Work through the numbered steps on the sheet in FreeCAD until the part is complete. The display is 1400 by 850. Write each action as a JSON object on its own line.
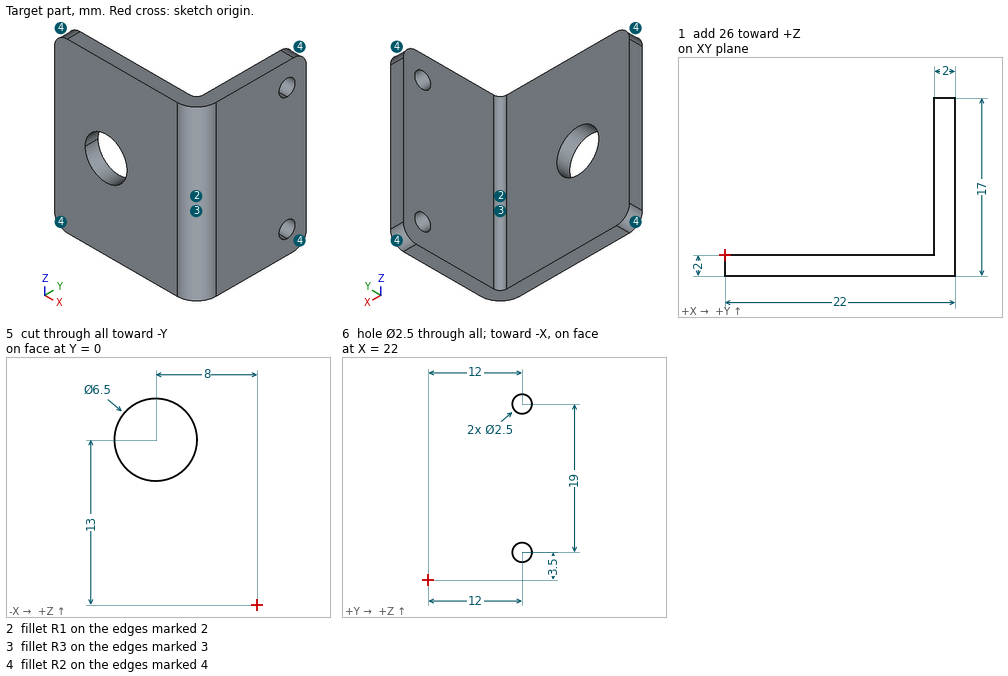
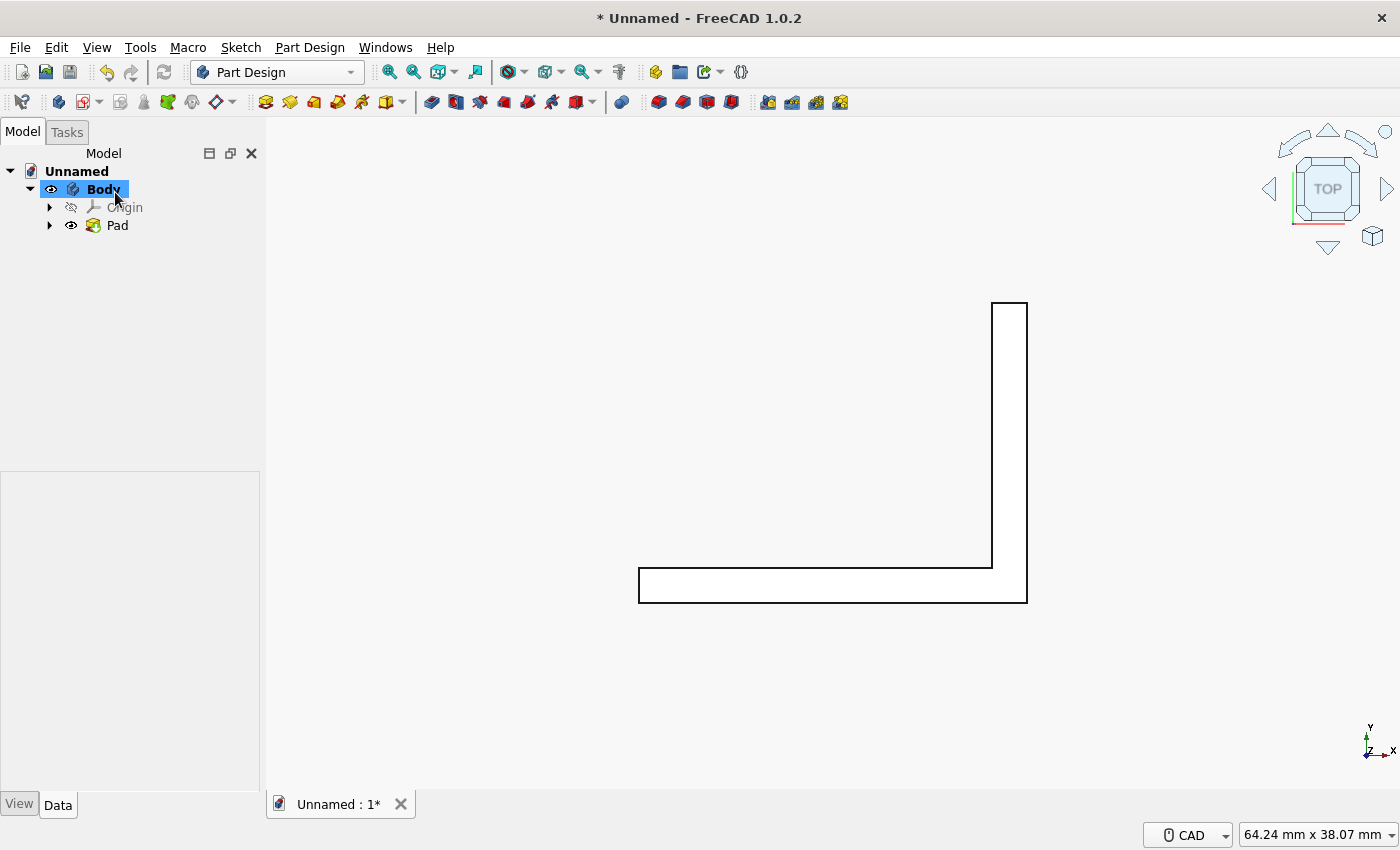
{"action": "key", "text": "v f"}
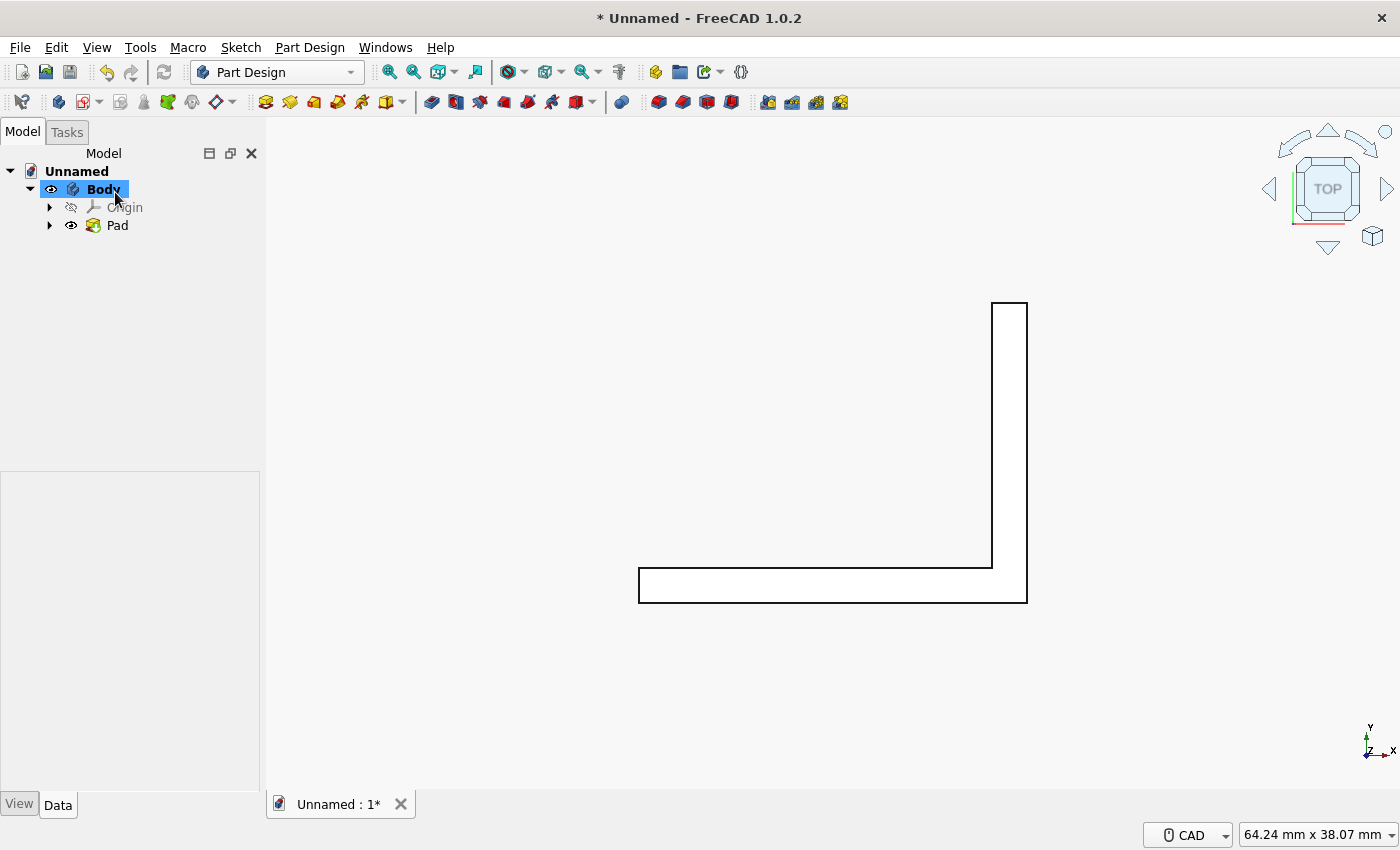
{"action": "key", "text": "1"}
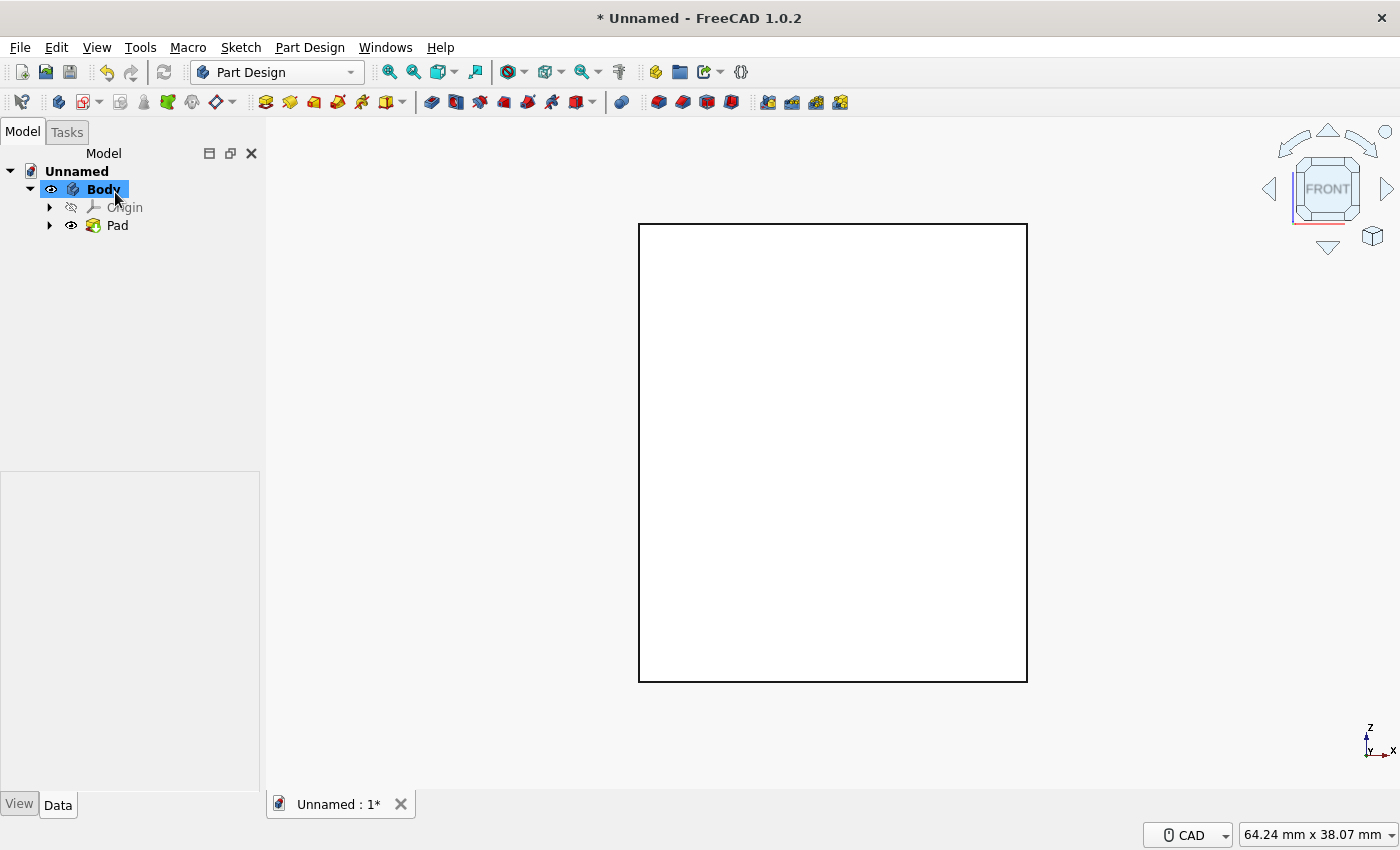
{"action": "key", "text": "3"}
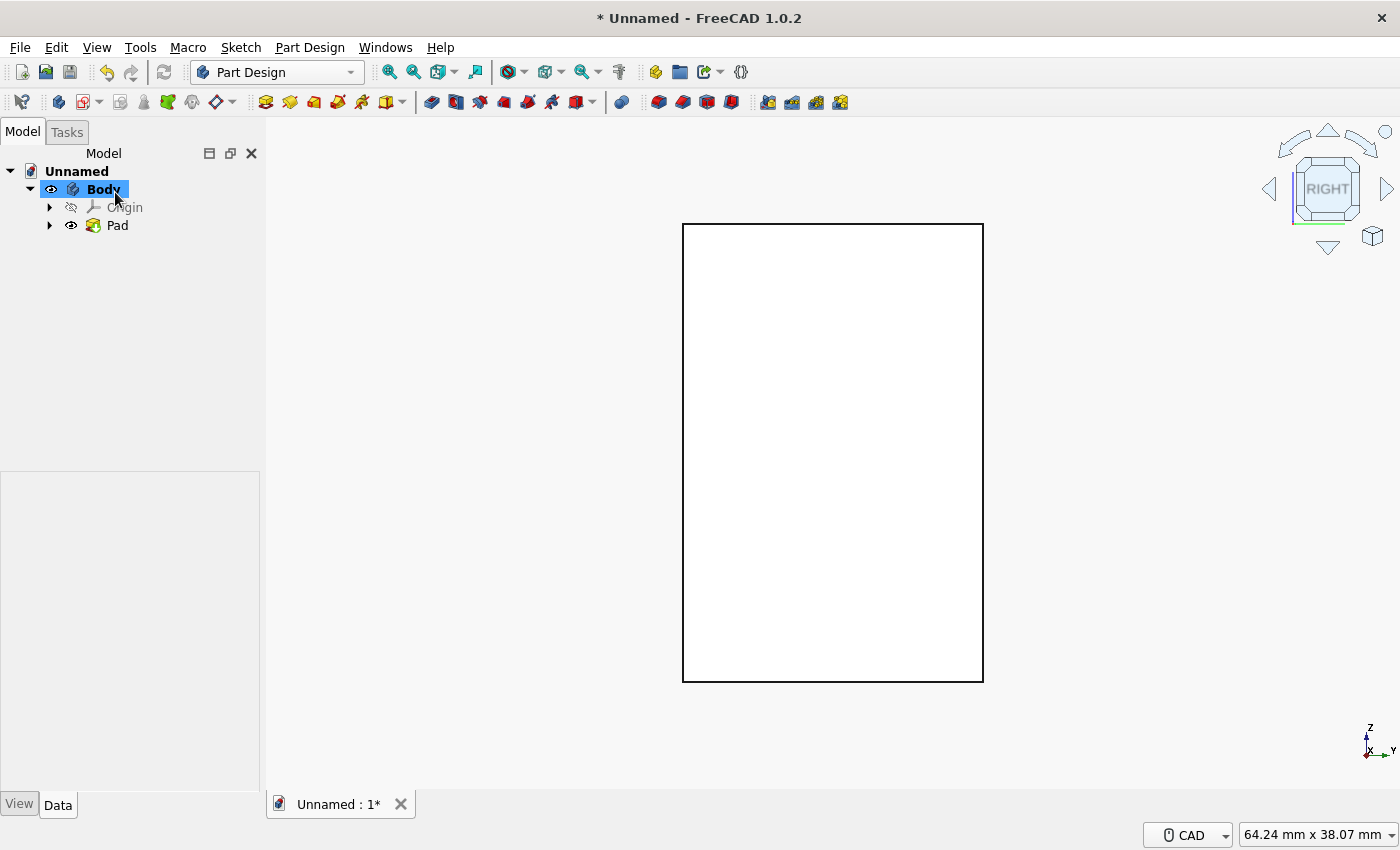
{"action": "key", "text": "5"}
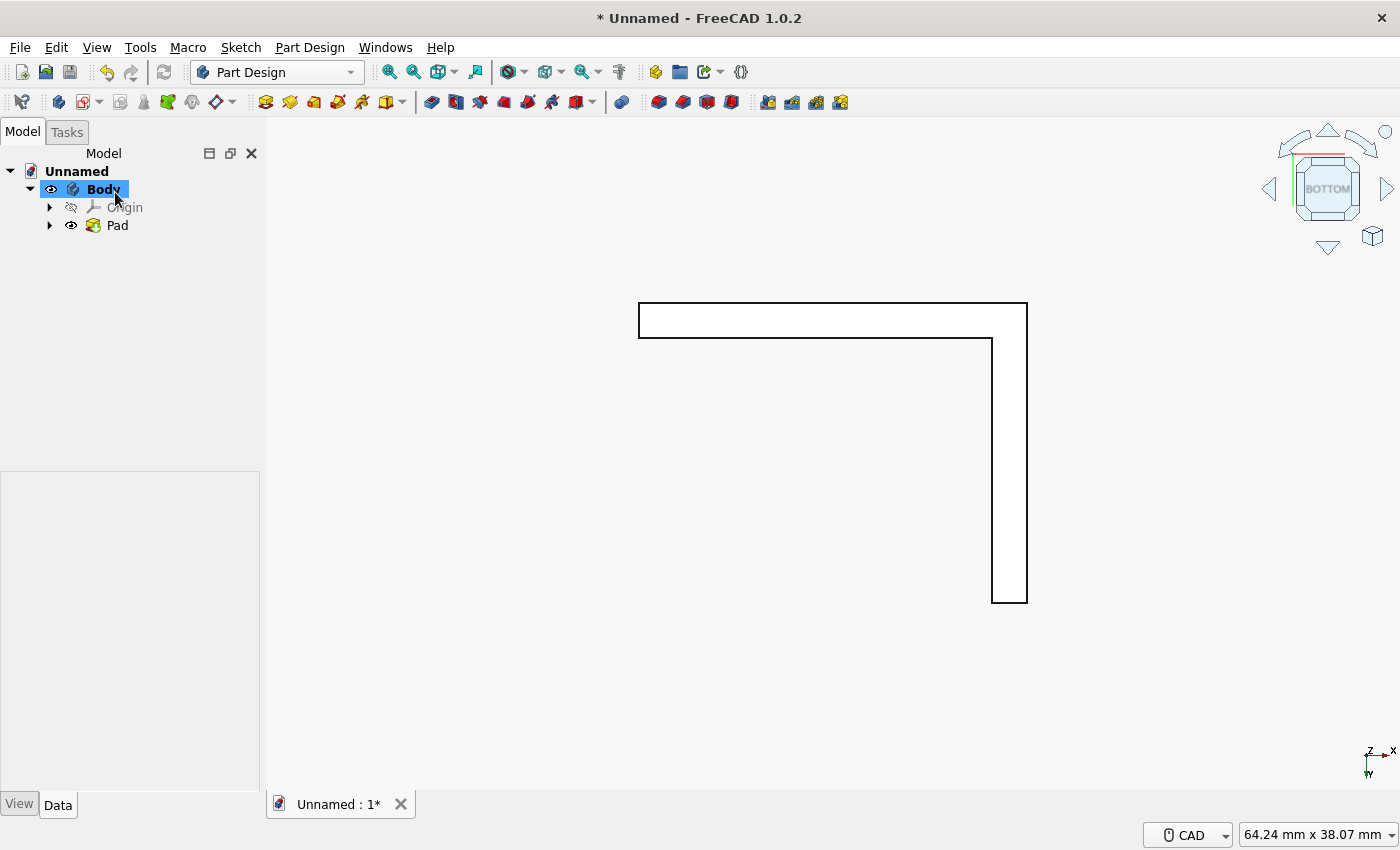
{"action": "key", "text": "v f"}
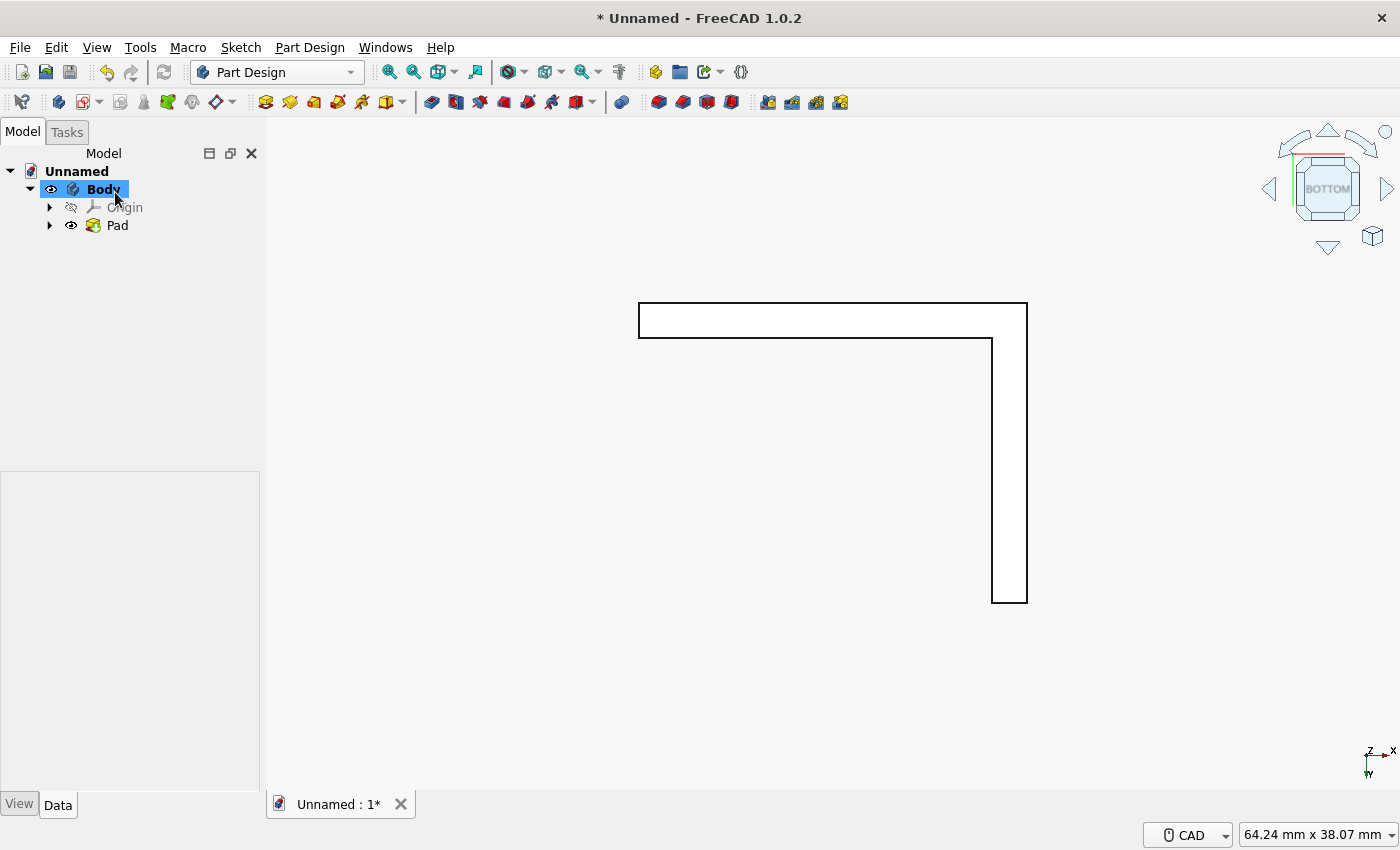
{"action": "key", "text": "4"}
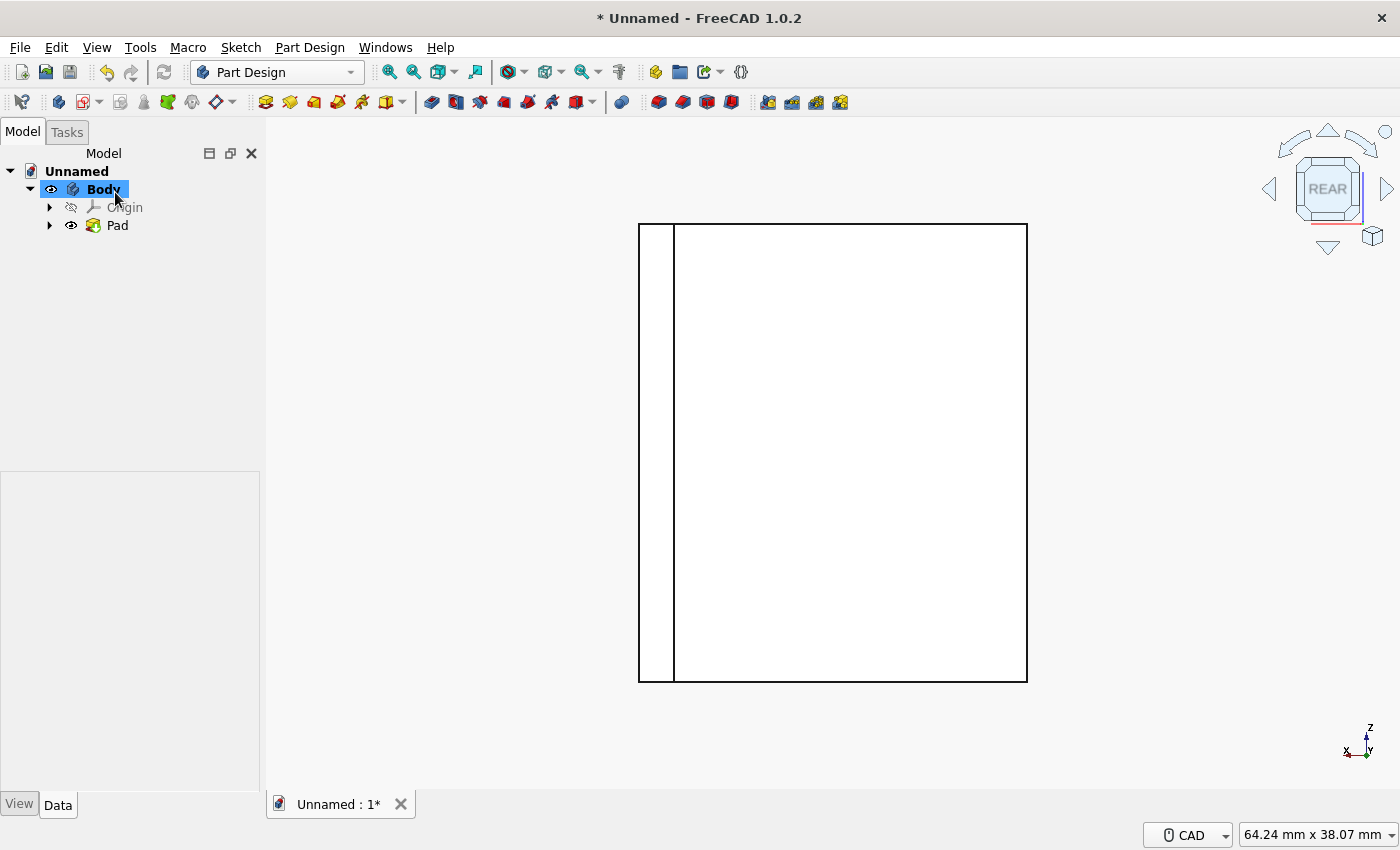
{"action": "key", "text": "6"}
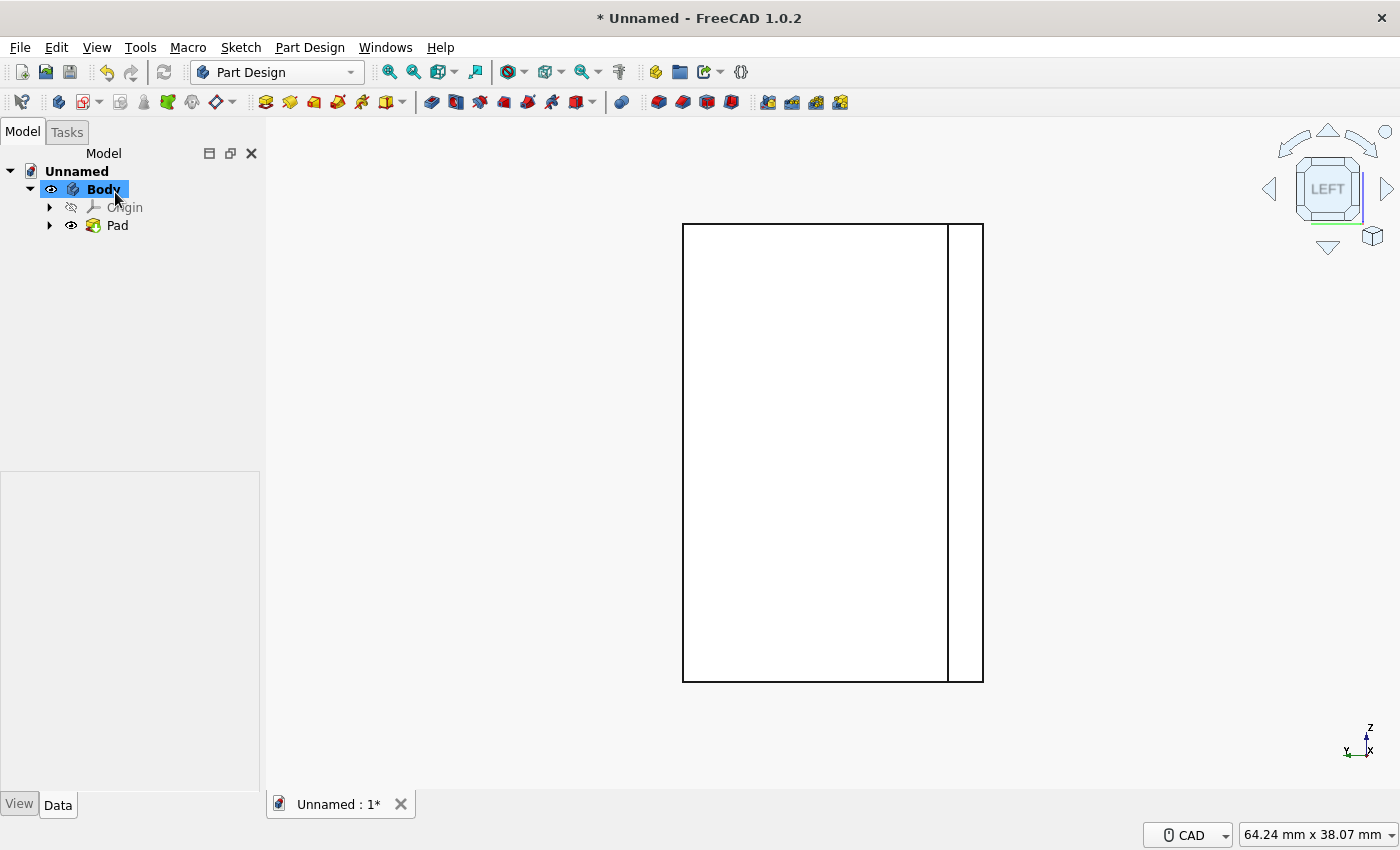
{"action": "key", "text": "v 3"}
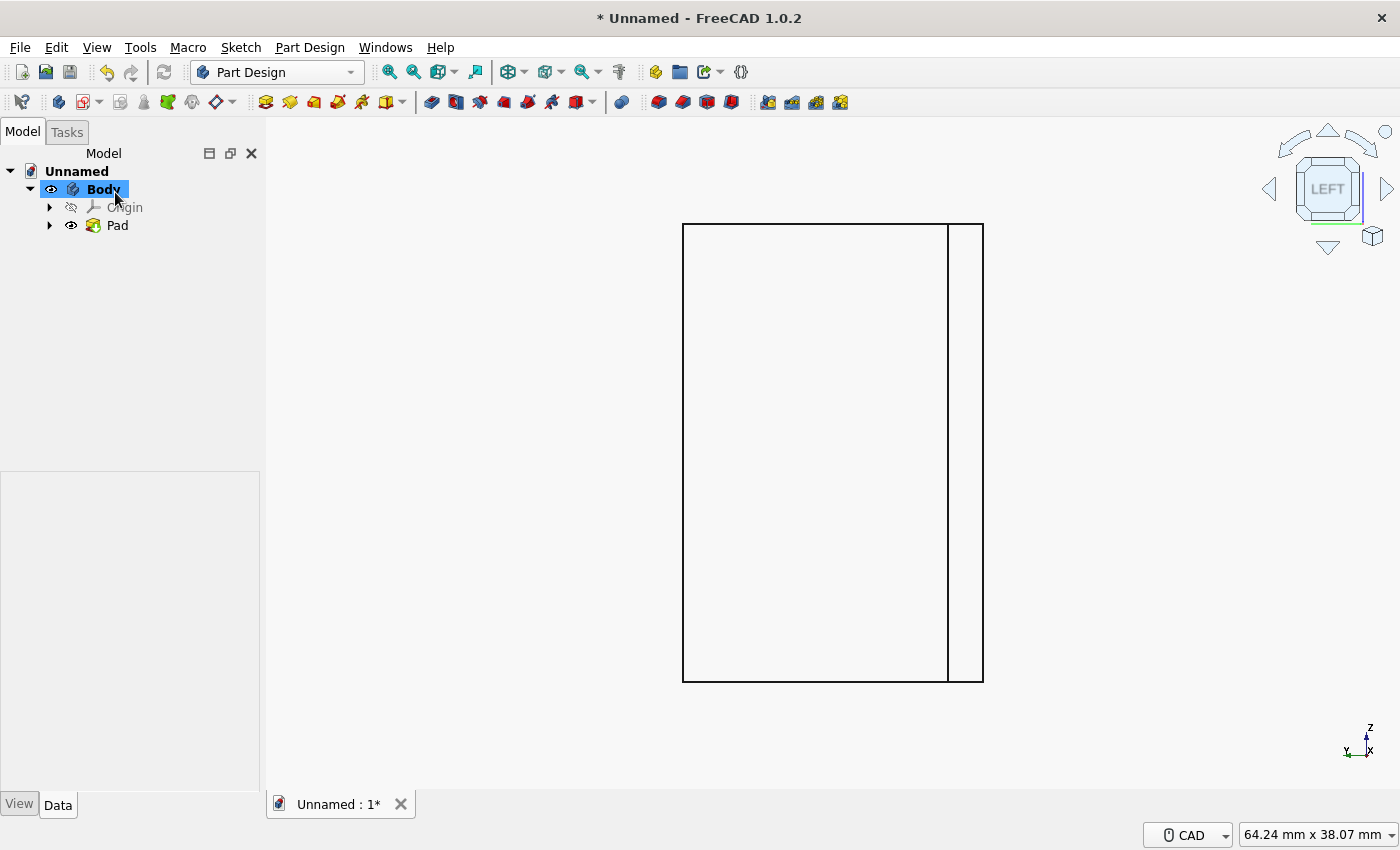
{"action": "key", "text": "0"}